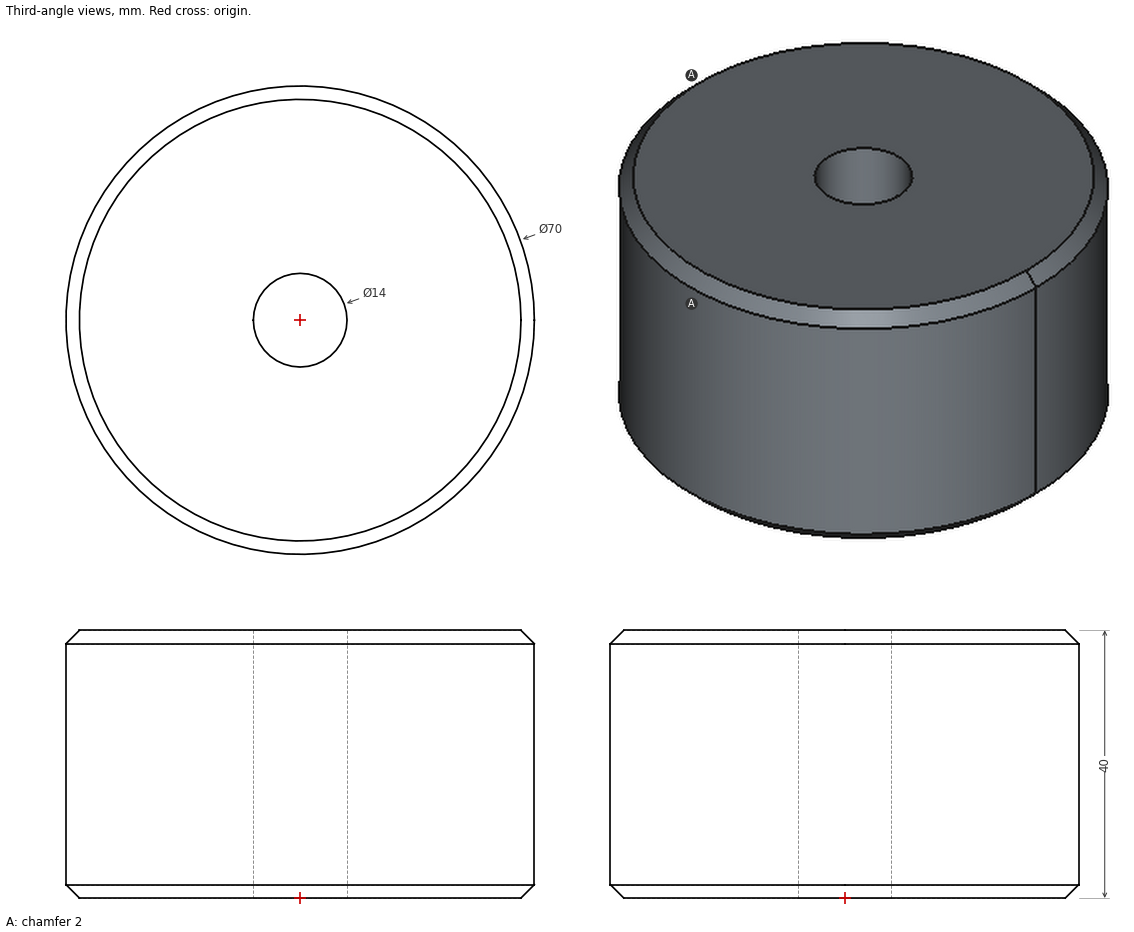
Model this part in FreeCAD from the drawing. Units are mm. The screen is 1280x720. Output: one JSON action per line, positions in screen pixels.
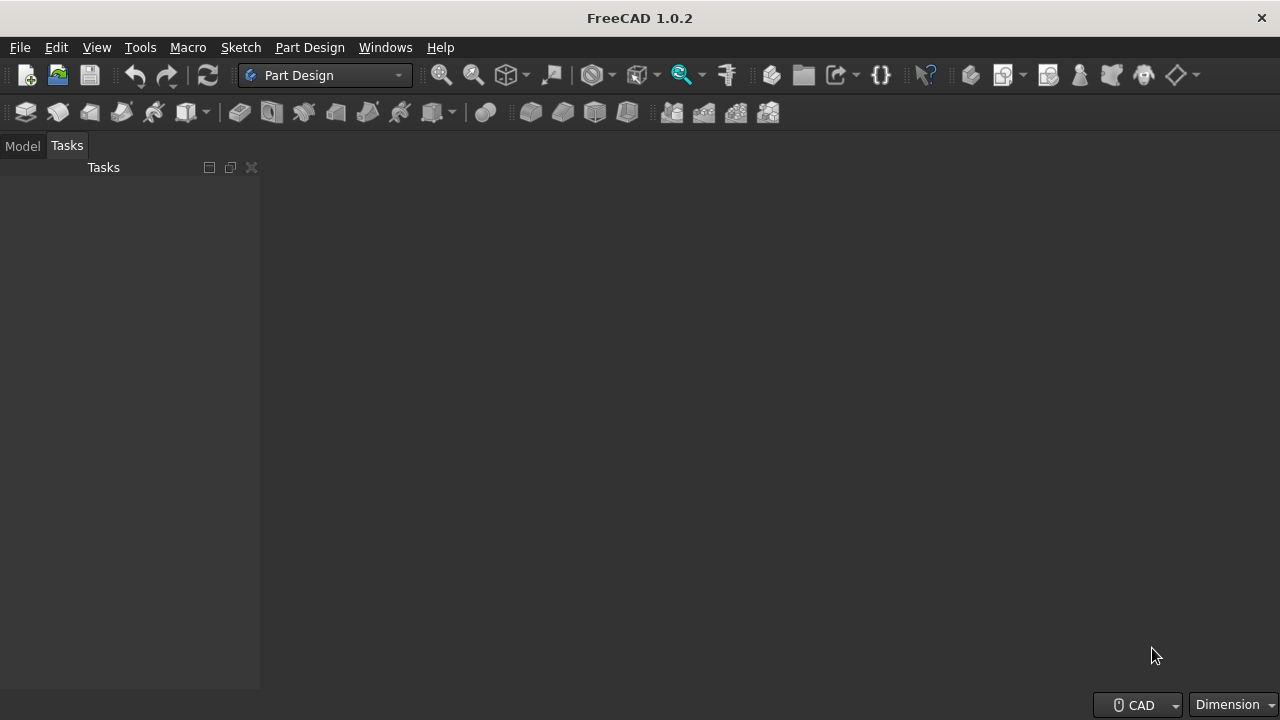
{"action": "key", "text": "ctrl+n"}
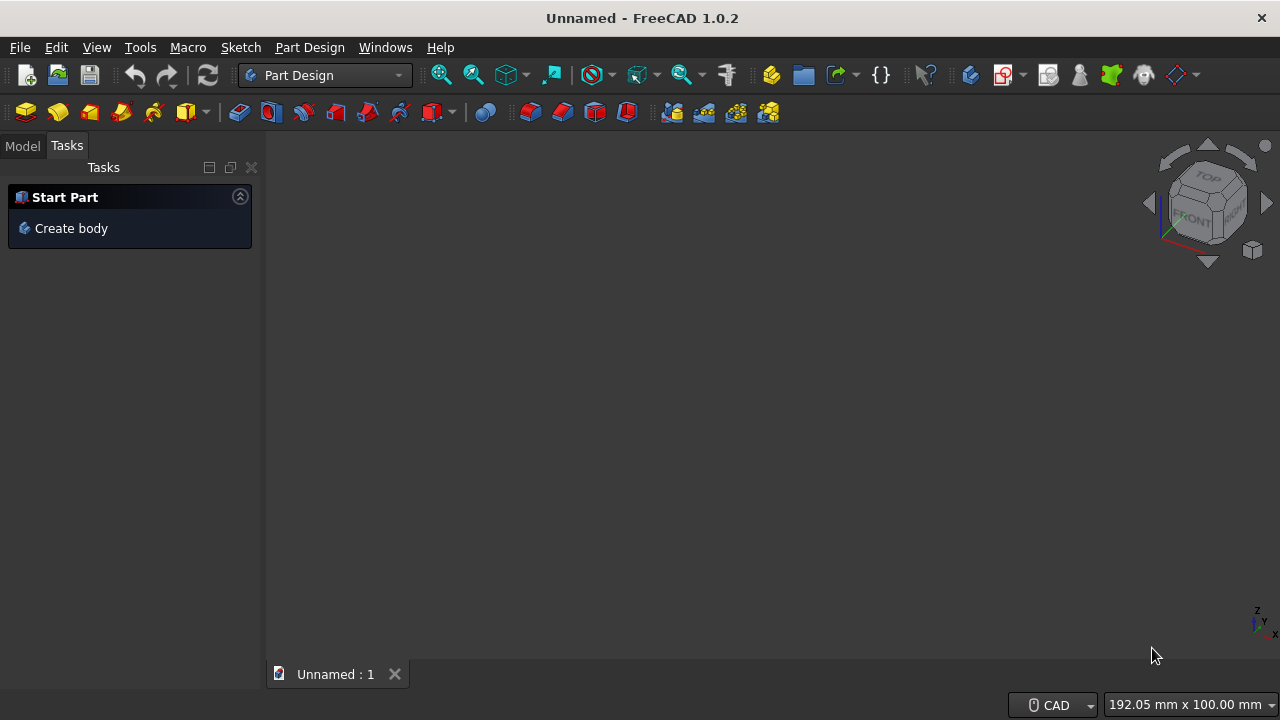
{"action": "left_click", "coordinate": [1004, 76]}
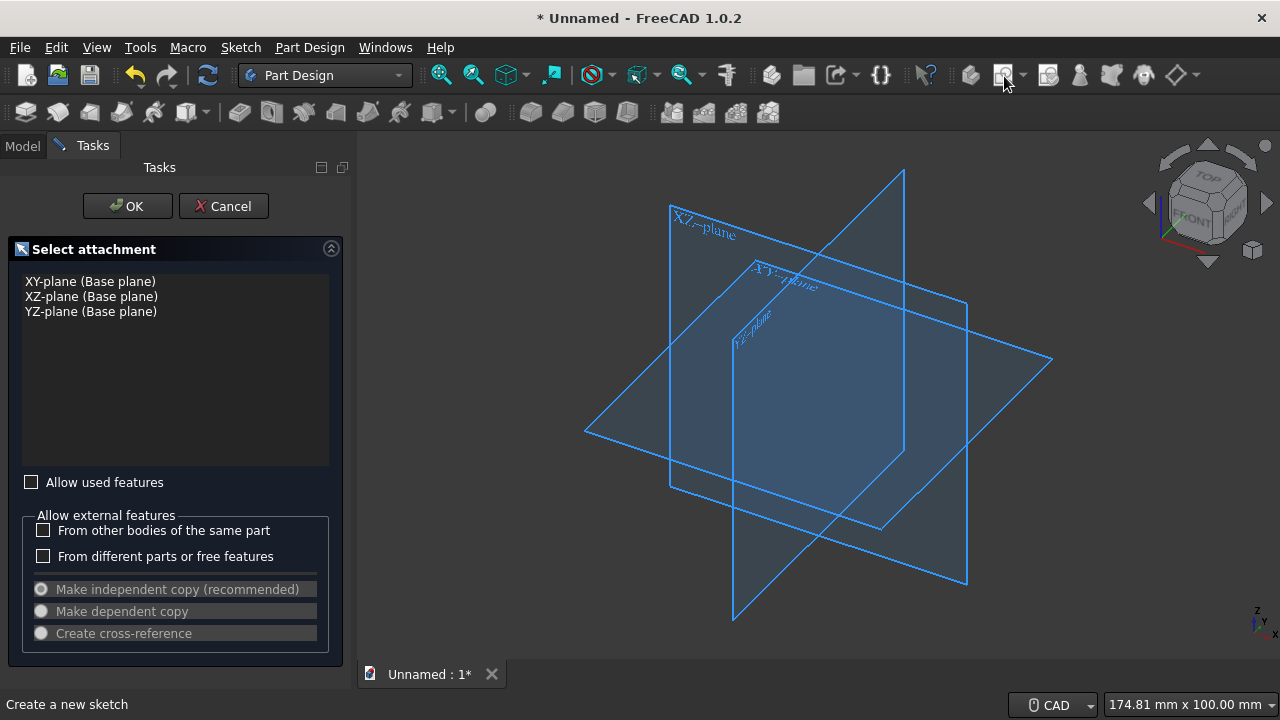
{"action": "left_click", "coordinate": [82, 282]}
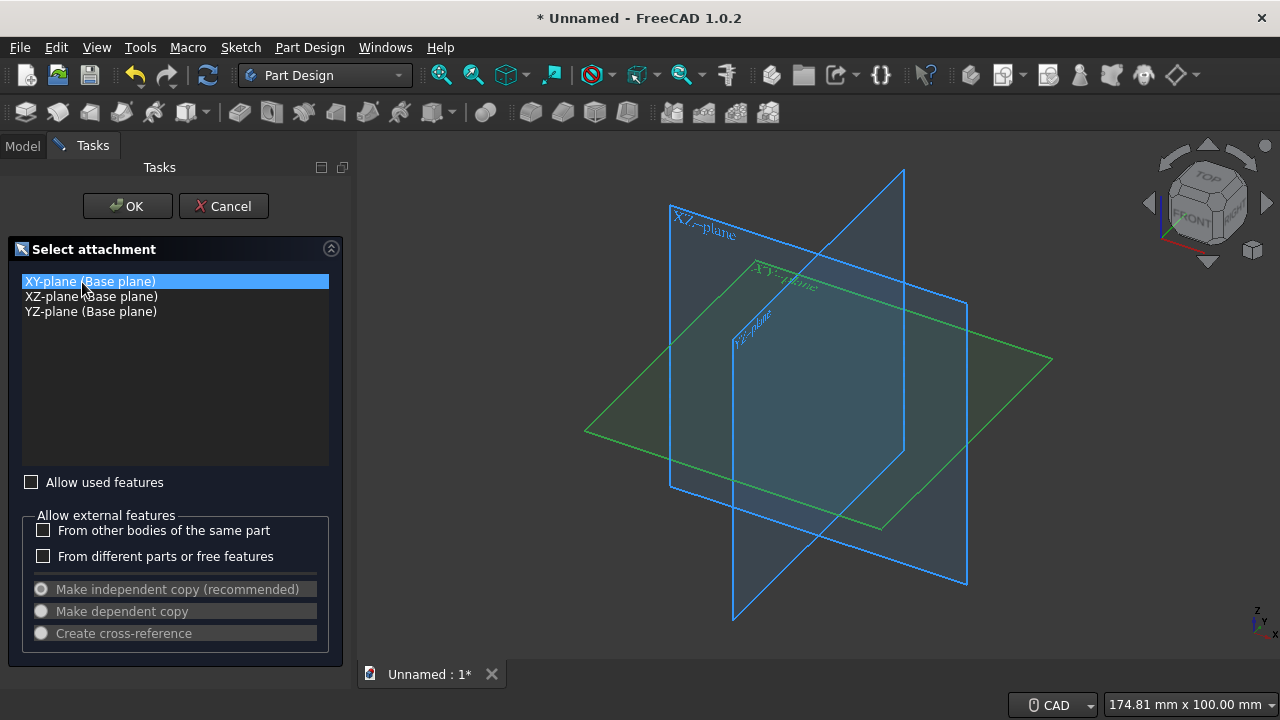
{"action": "left_click", "coordinate": [128, 206]}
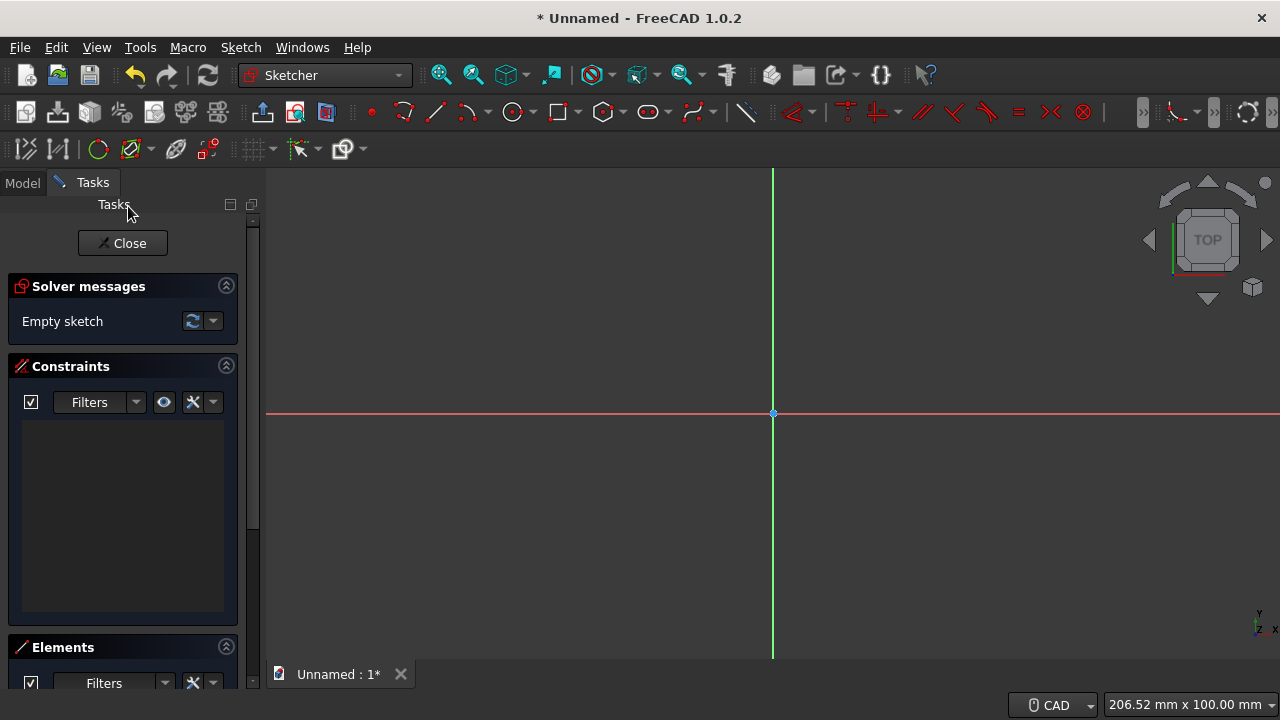
{"action": "key", "text": "g c"}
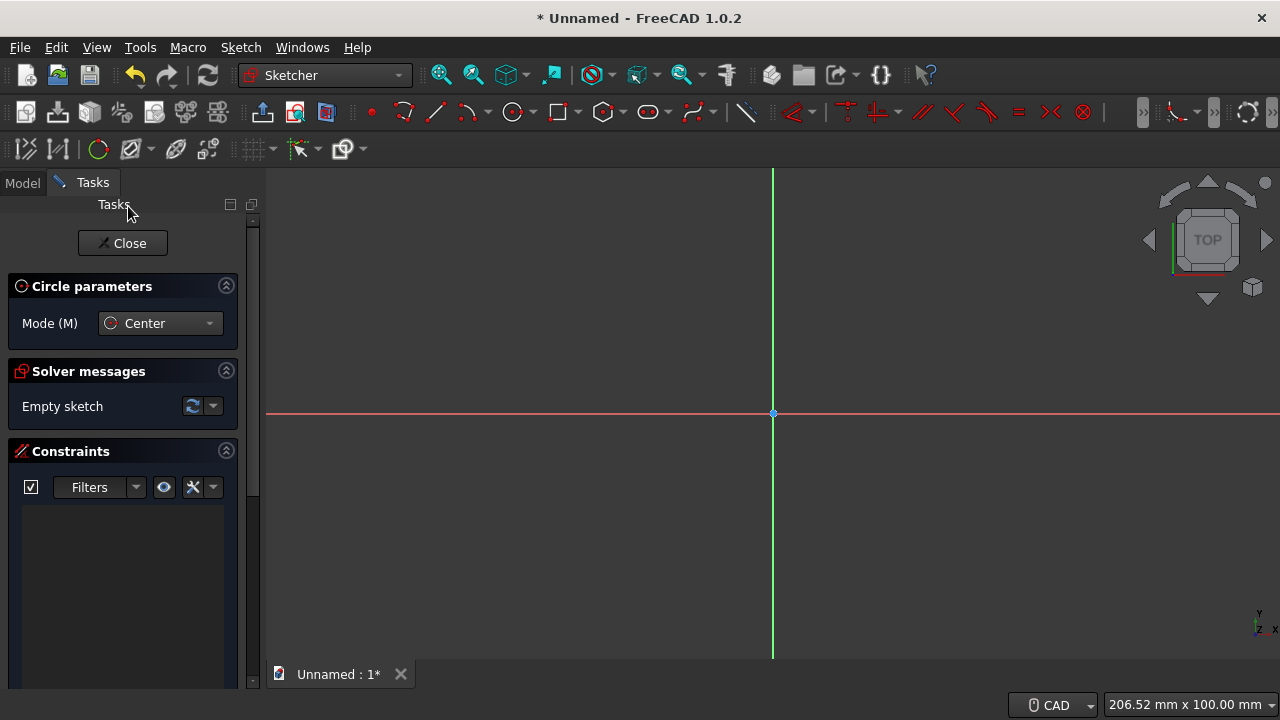
{"action": "left_click", "coordinate": [773, 414]}
{"action": "left_click", "coordinate": [895, 292]}
{"action": "key", "text": "Escape"}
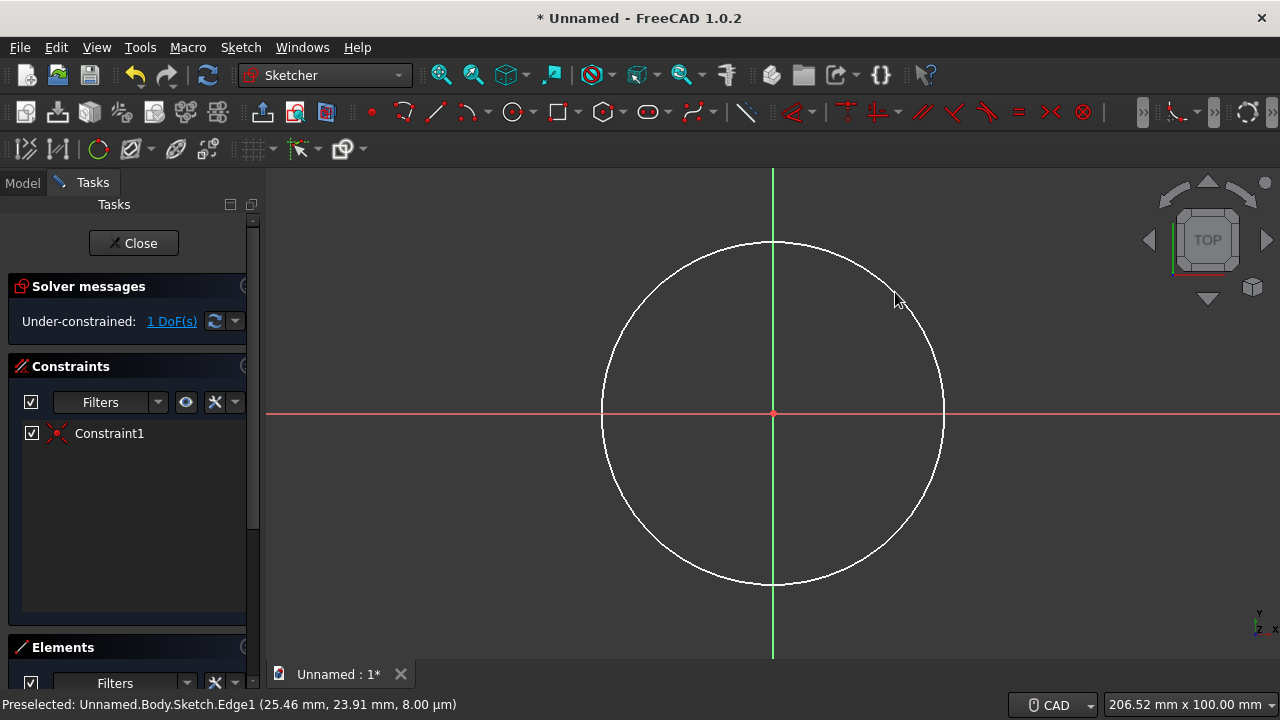
{"action": "left_click", "coordinate": [792, 112]}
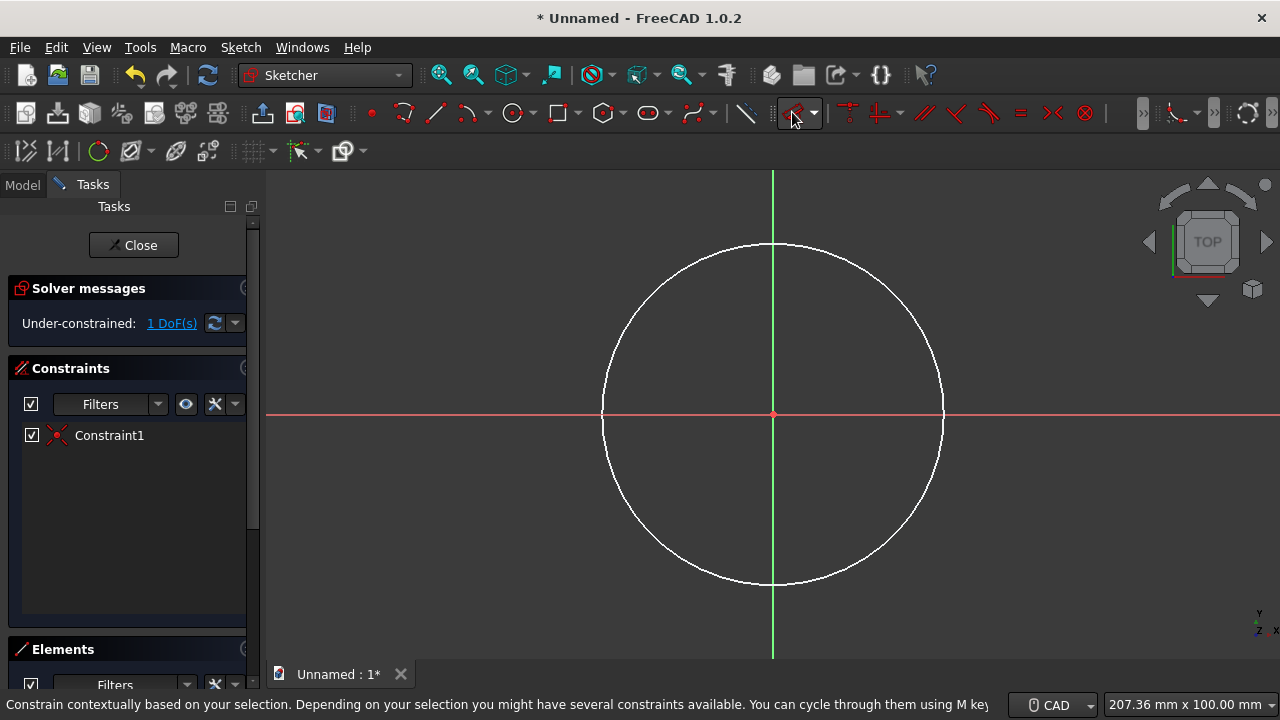
{"action": "left_click", "coordinate": [893, 293]}
{"action": "left_click", "coordinate": [915, 270]}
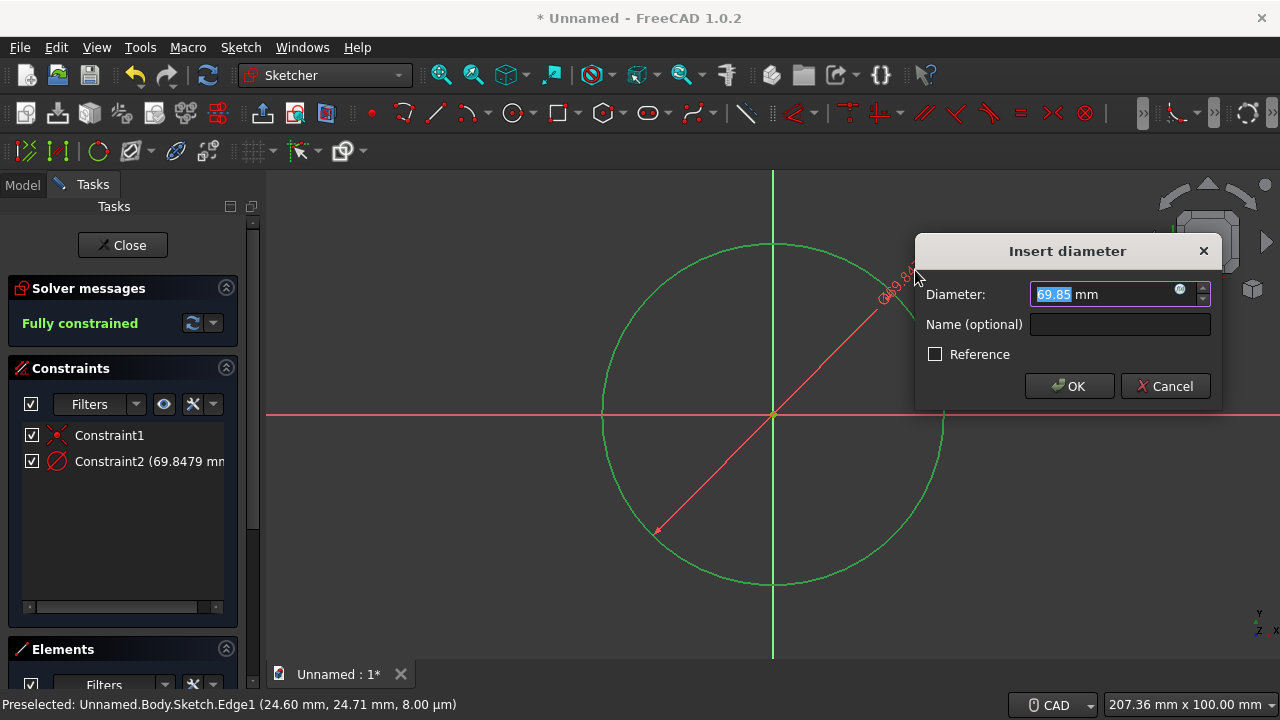
{"action": "type", "text": "70"}
{"action": "key", "text": "Return"}
{"action": "key", "text": "Escape"}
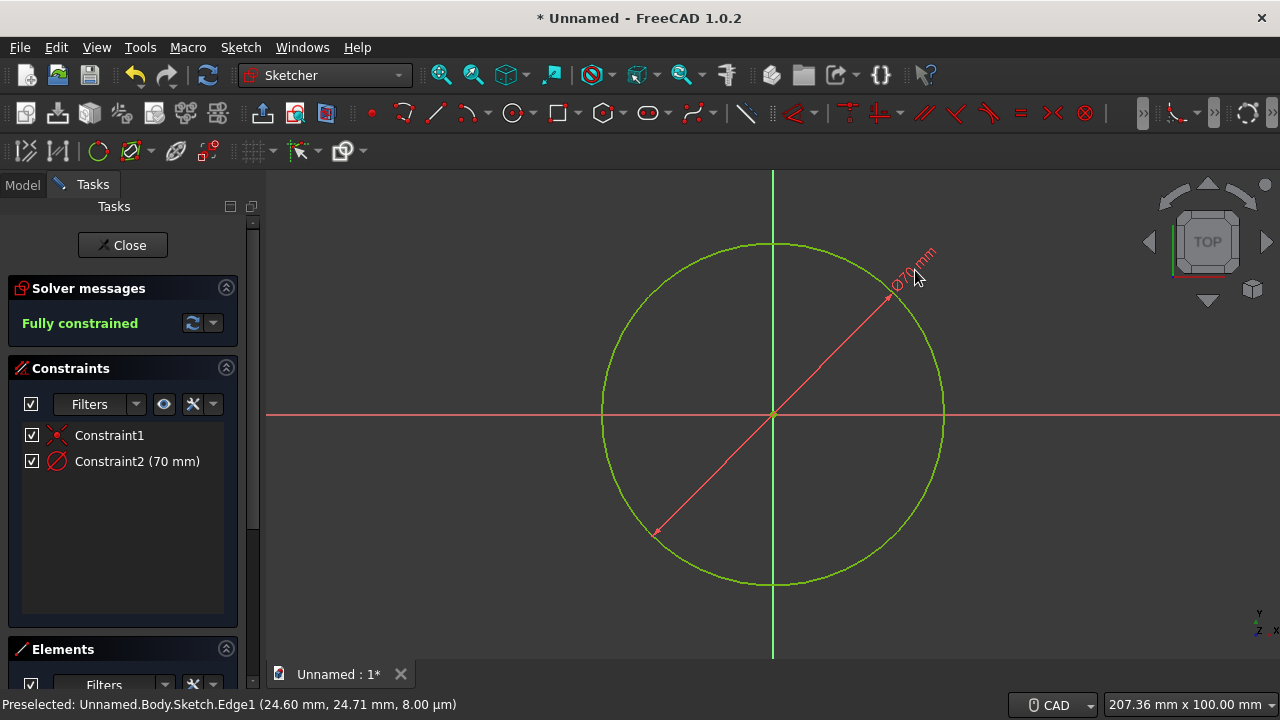
{"action": "left_click", "coordinate": [123, 245]}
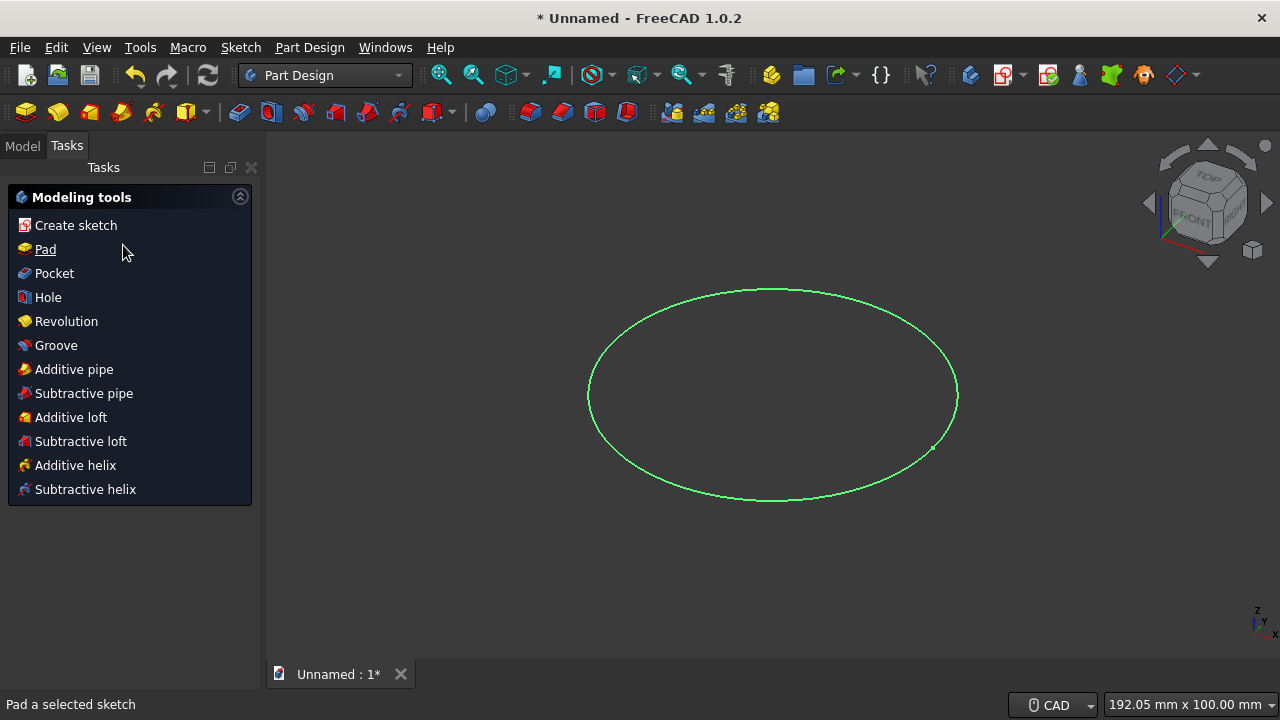
{"action": "left_click", "coordinate": [26, 112]}